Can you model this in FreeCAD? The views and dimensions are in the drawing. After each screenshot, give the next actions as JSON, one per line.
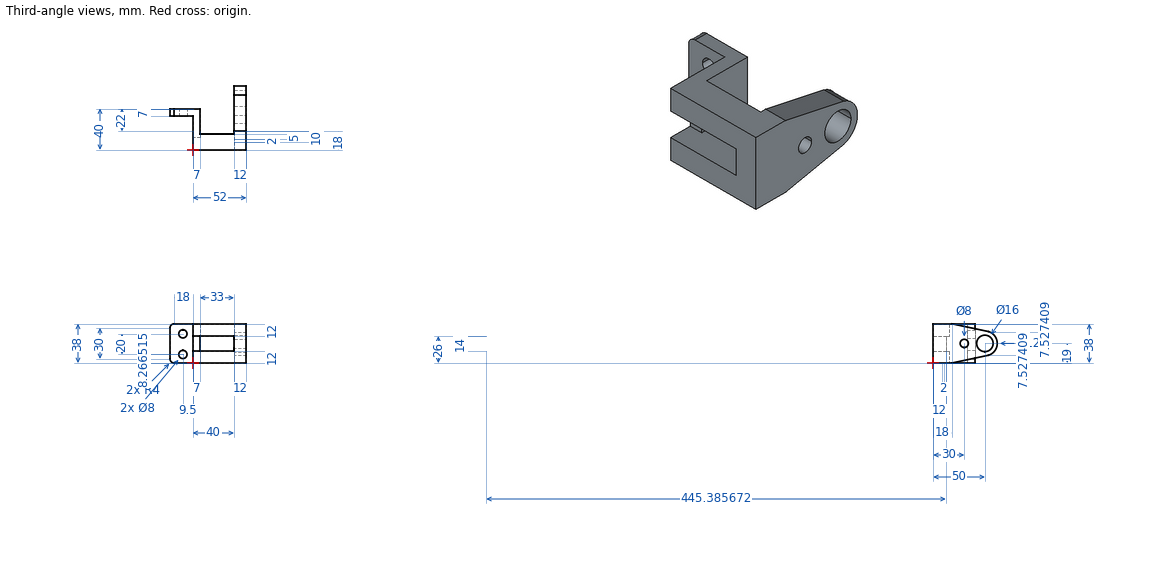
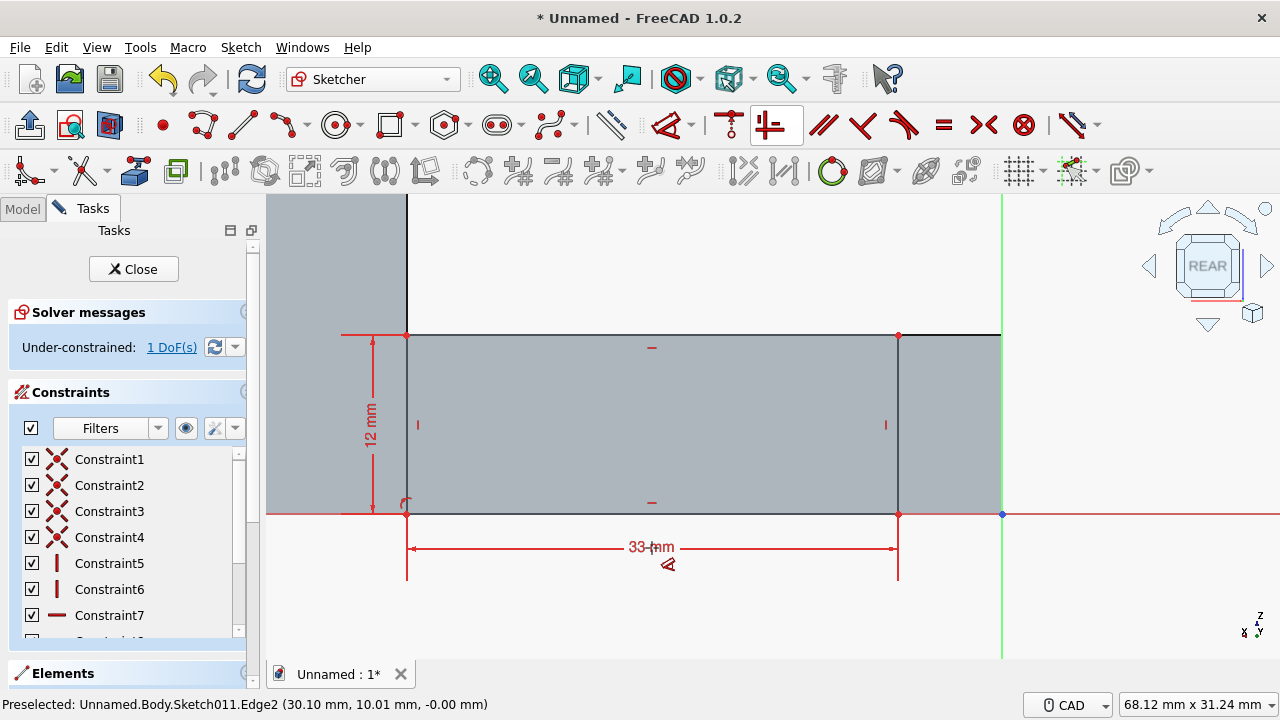
{"action": "left_click", "coordinate": [898, 514]}
{"action": "left_click", "coordinate": [950, 548]}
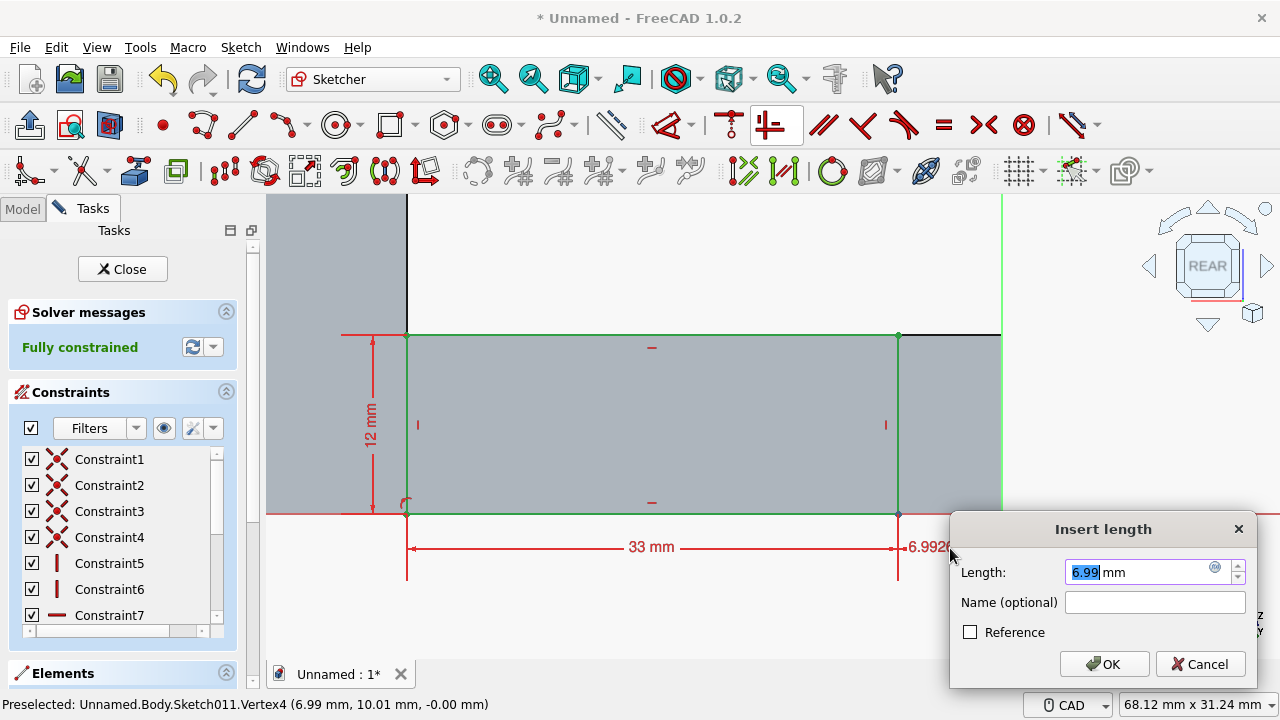
{"action": "type", "text": "7"}
{"action": "key", "text": "Return"}
{"action": "key", "text": "Escape"}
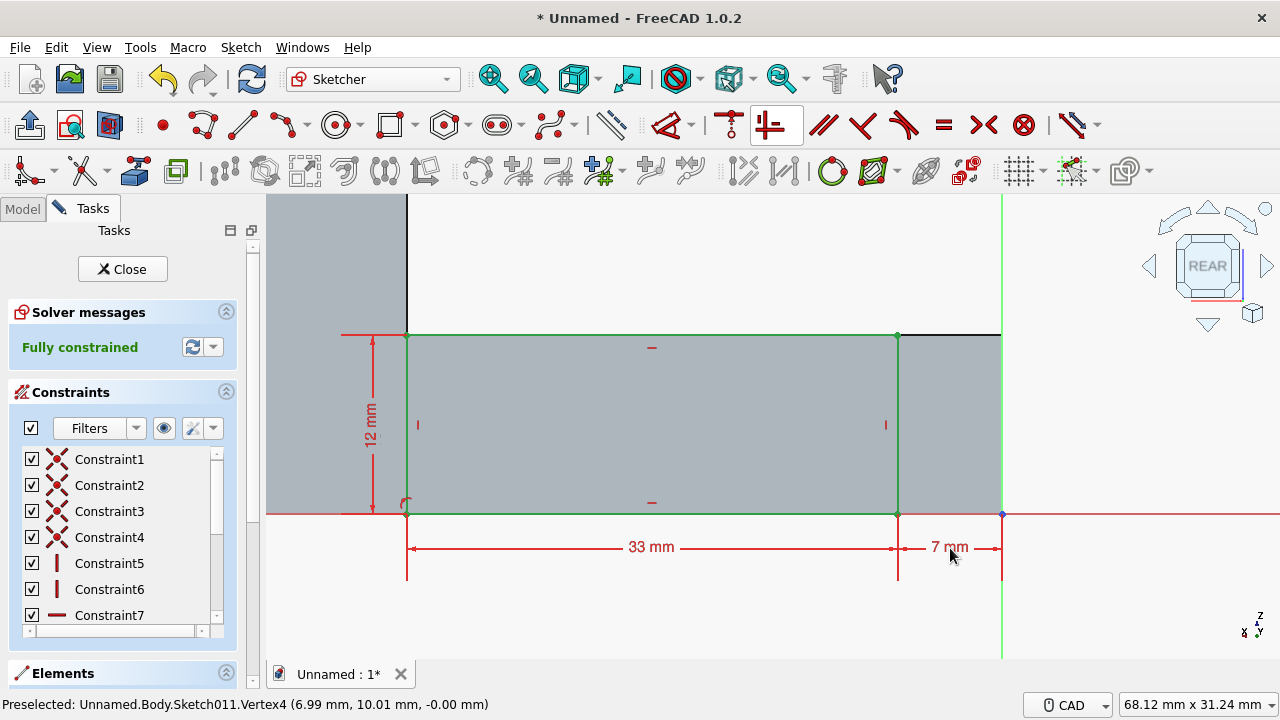
{"action": "left_click", "coordinate": [123, 269]}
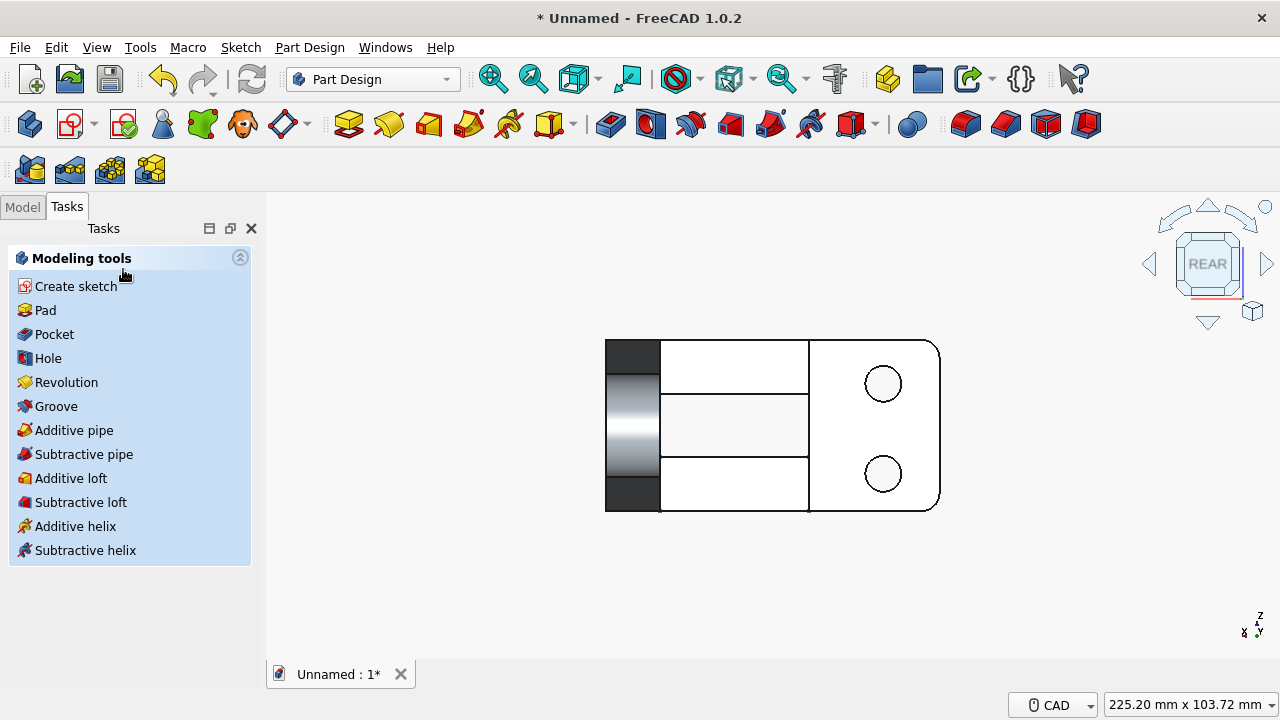
{"action": "left_click", "coordinate": [350, 124]}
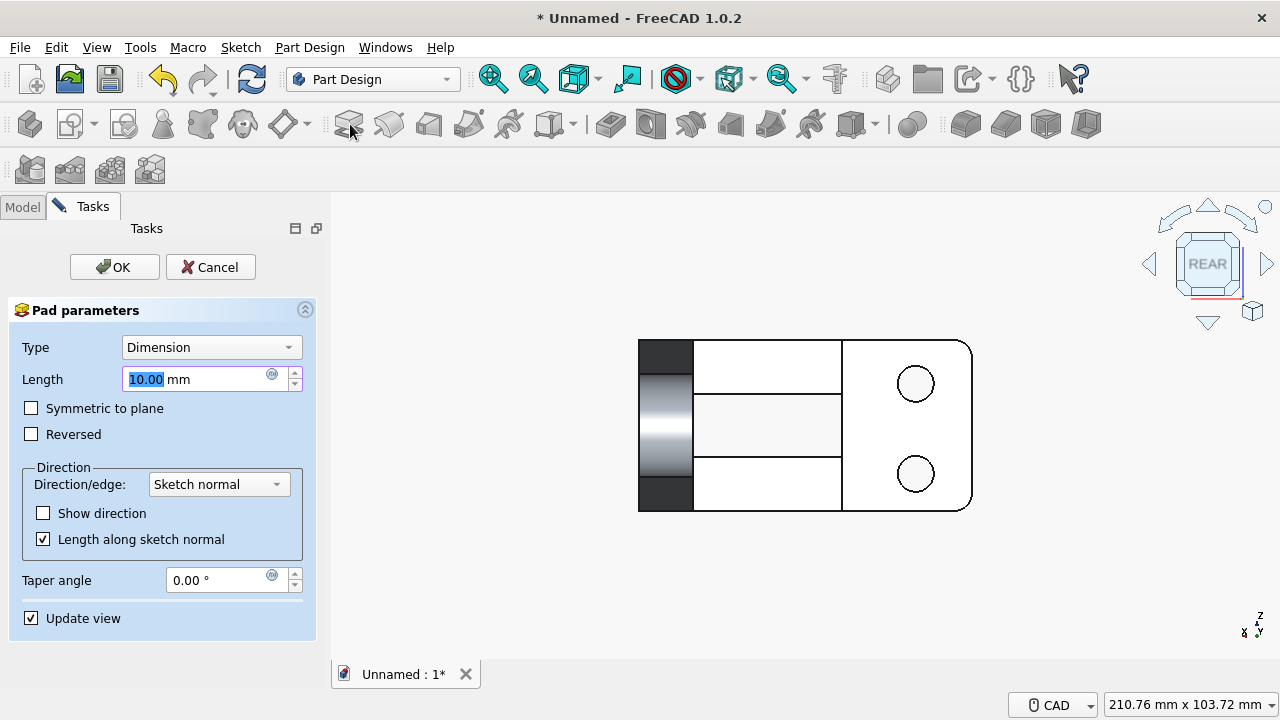
{"action": "type", "text": "5"}
{"action": "key", "text": "Tab"}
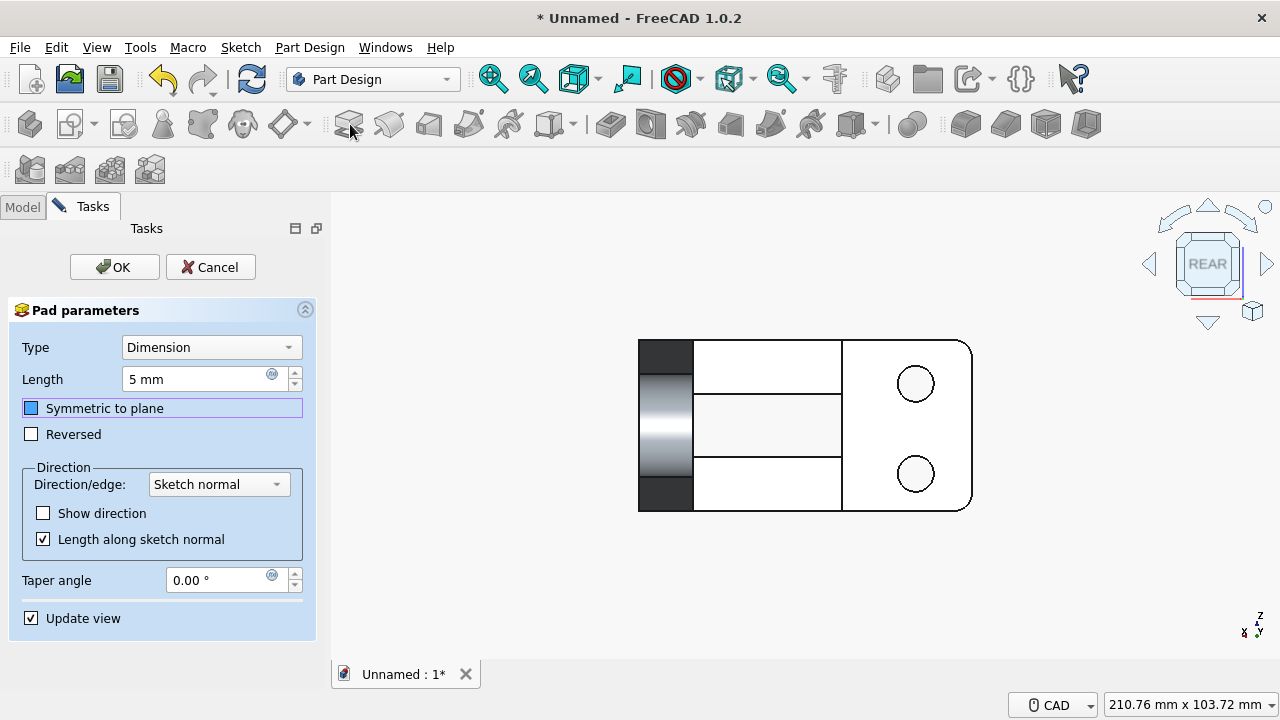
{"action": "left_click", "coordinate": [115, 267]}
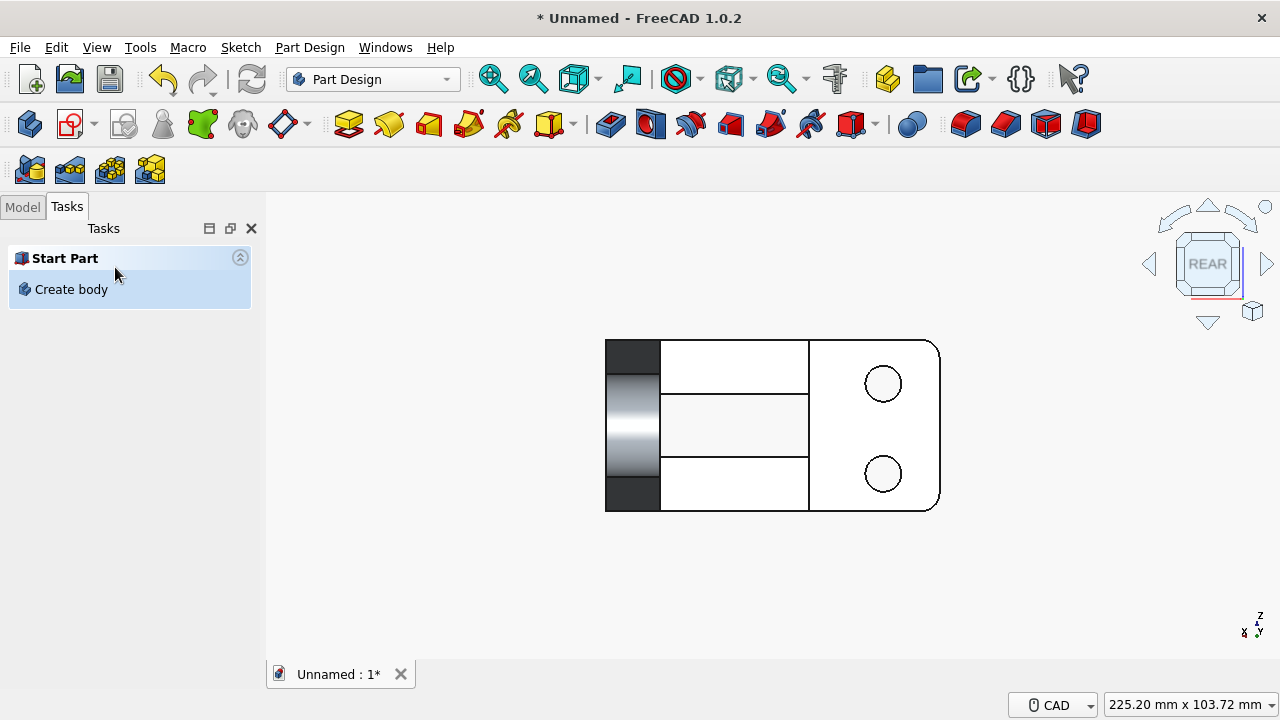
{"action": "key", "text": "0"}